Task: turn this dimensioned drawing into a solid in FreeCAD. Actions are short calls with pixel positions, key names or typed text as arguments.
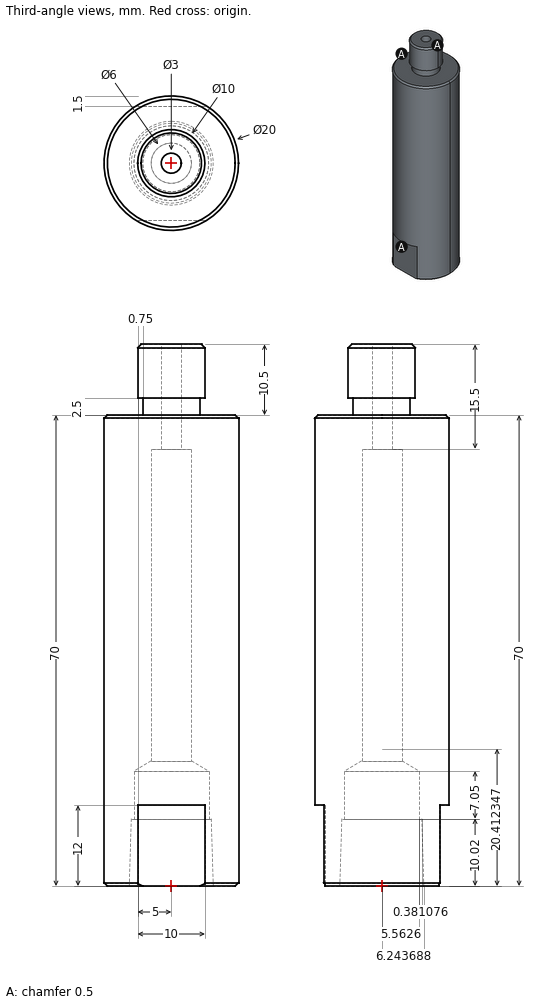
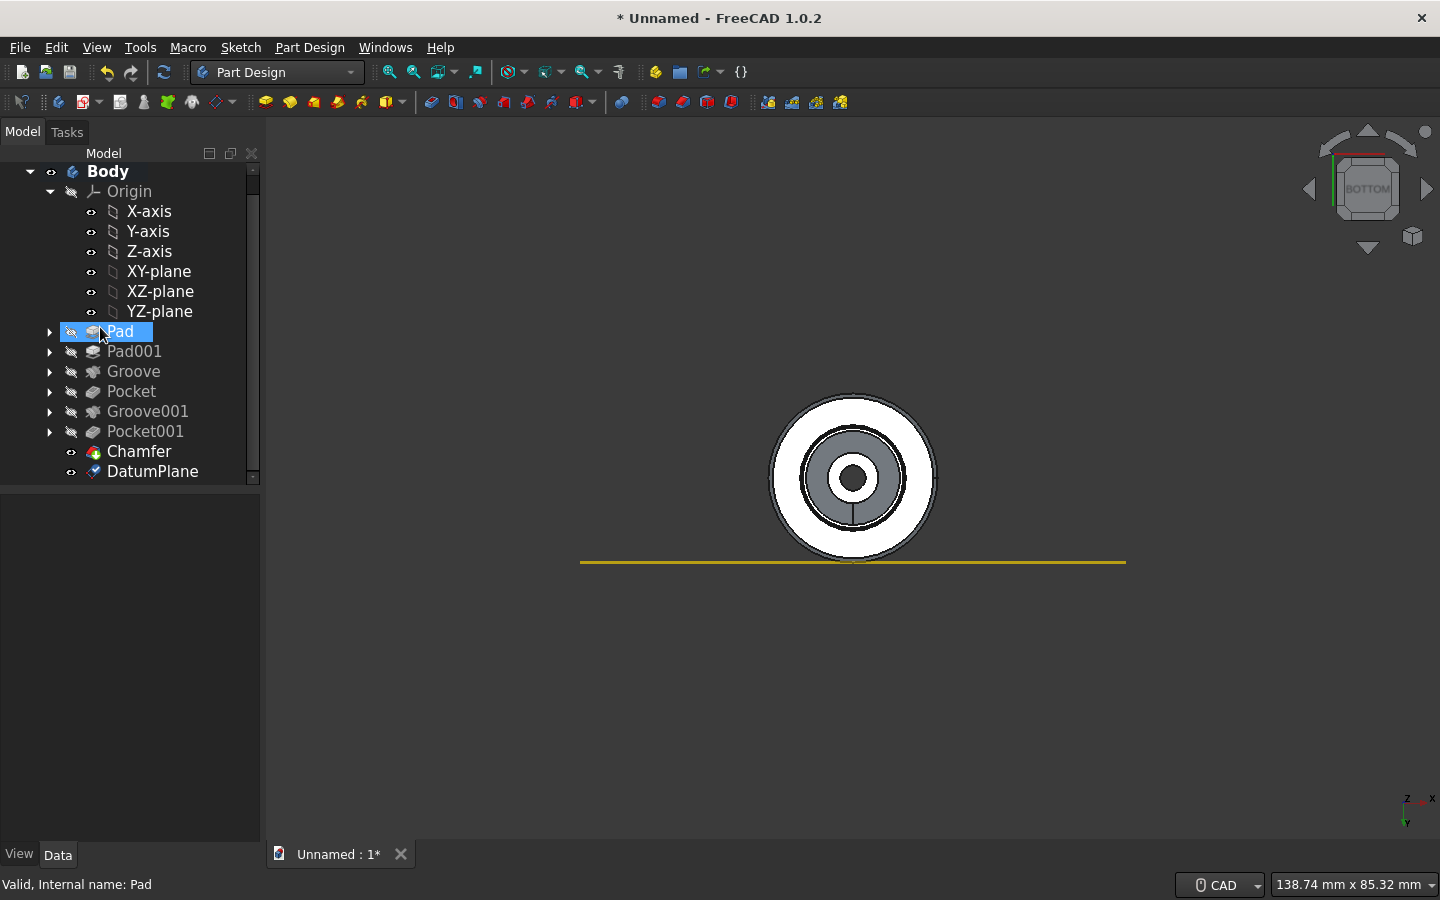
click(116, 472)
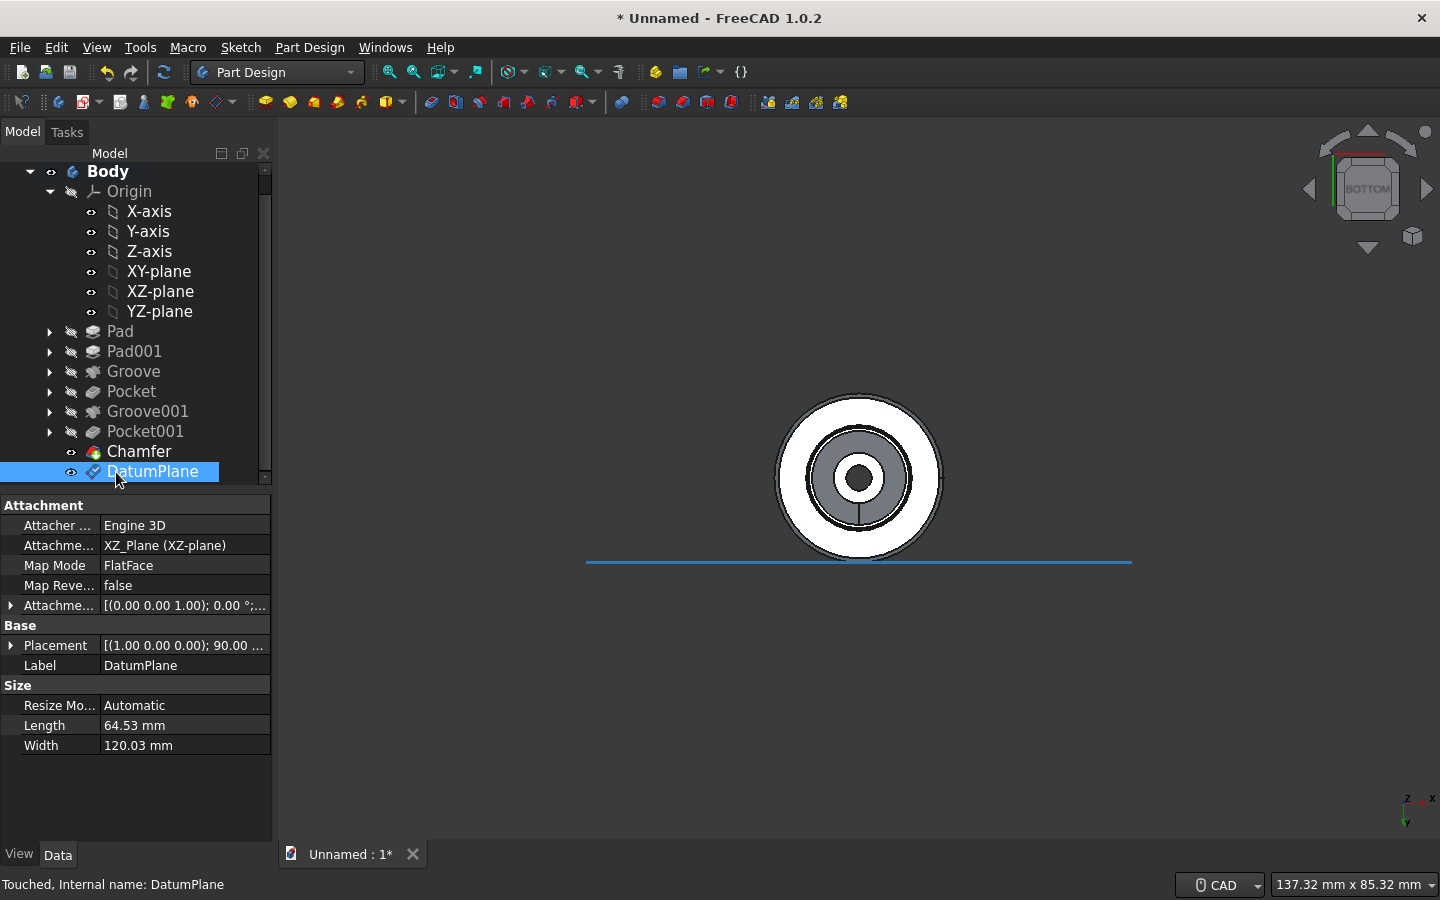
click(84, 102)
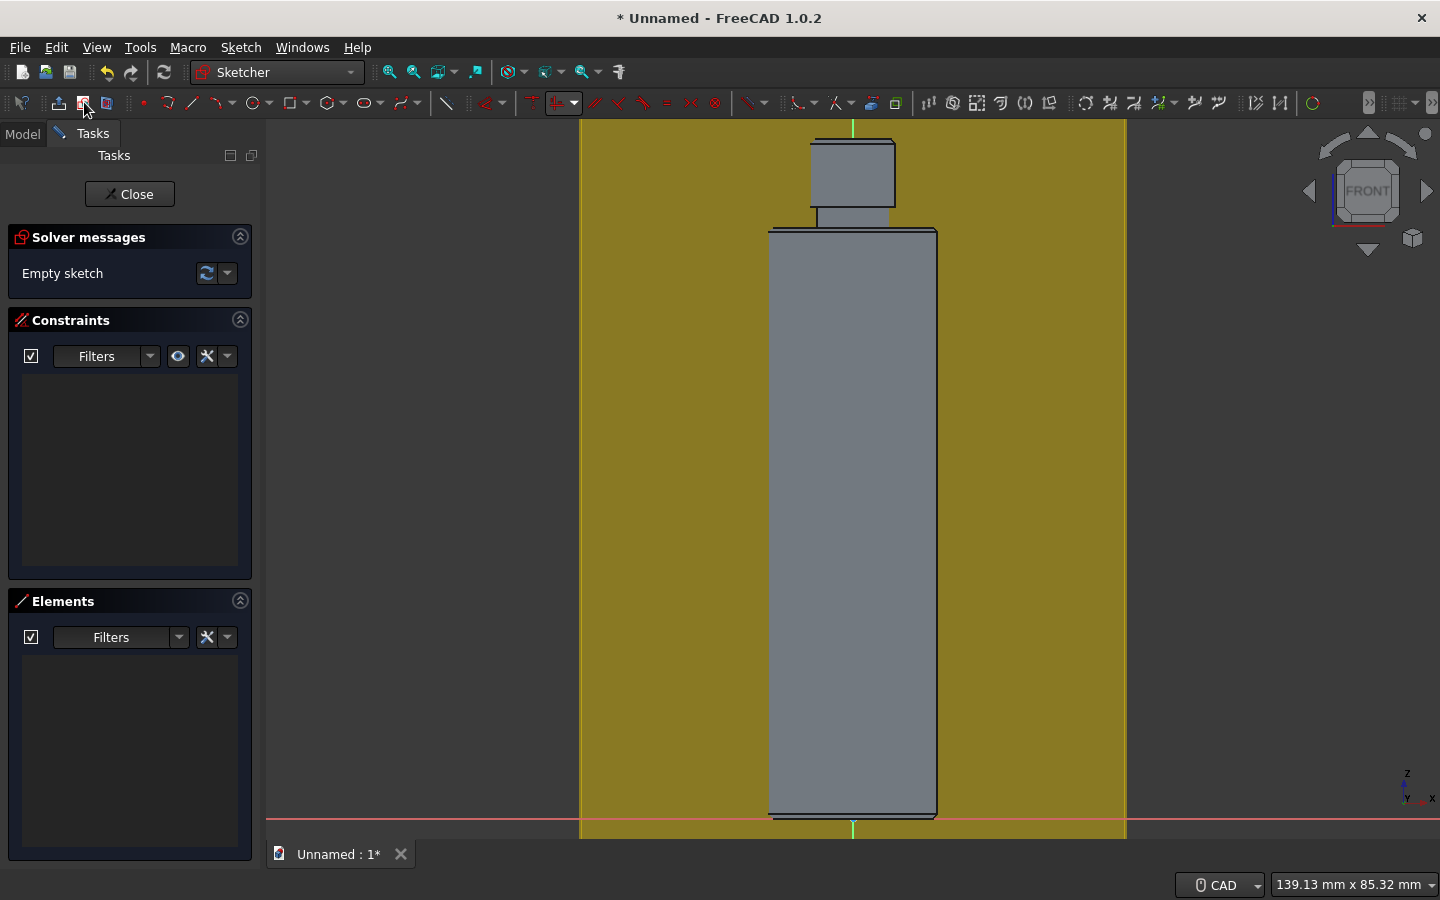
click(108, 104)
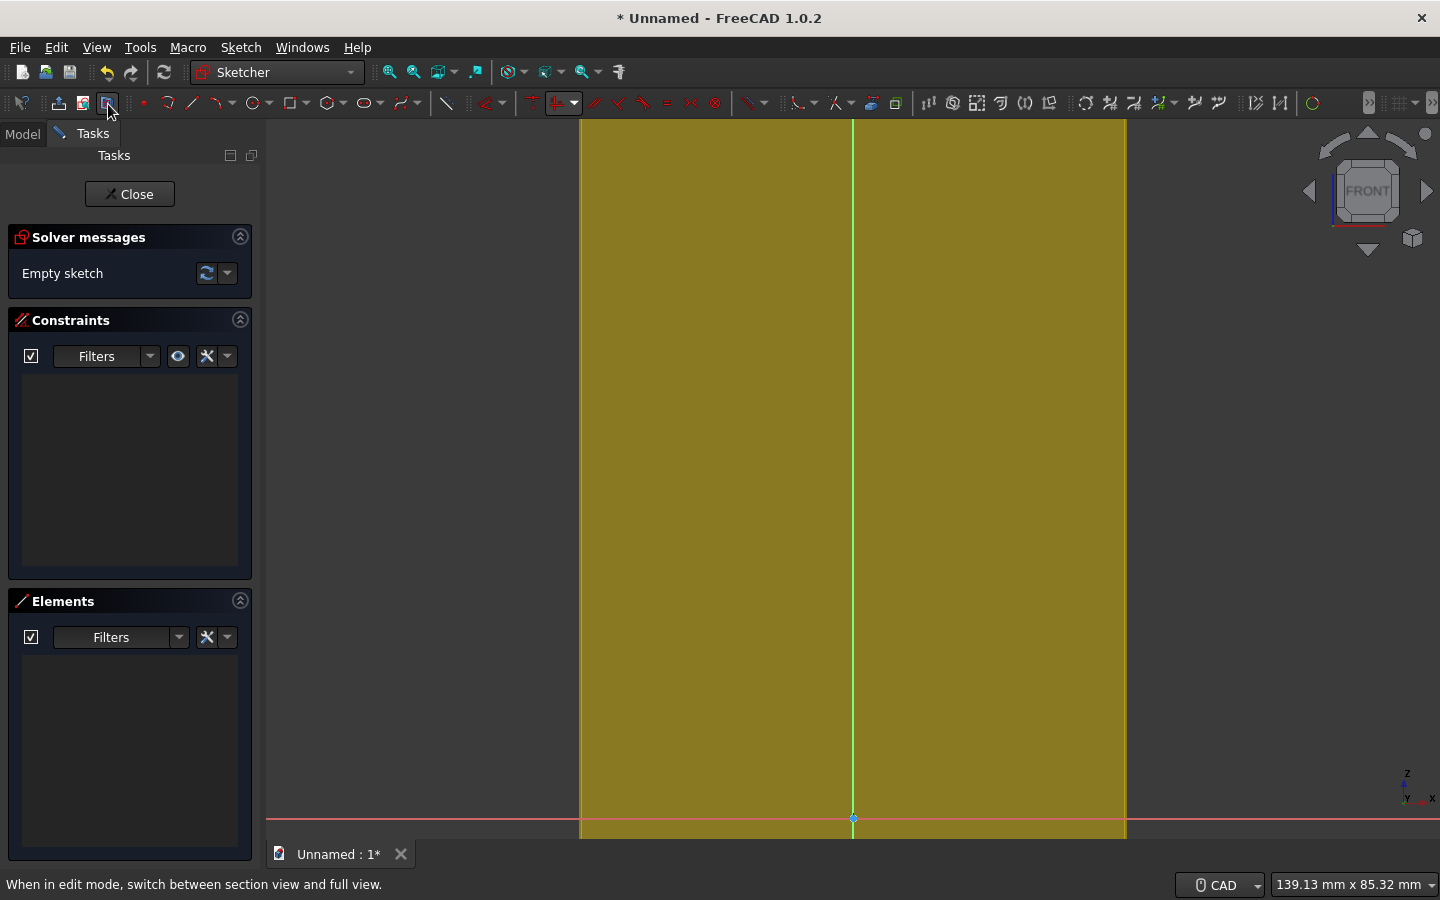
scroll(784, 479, down, 5)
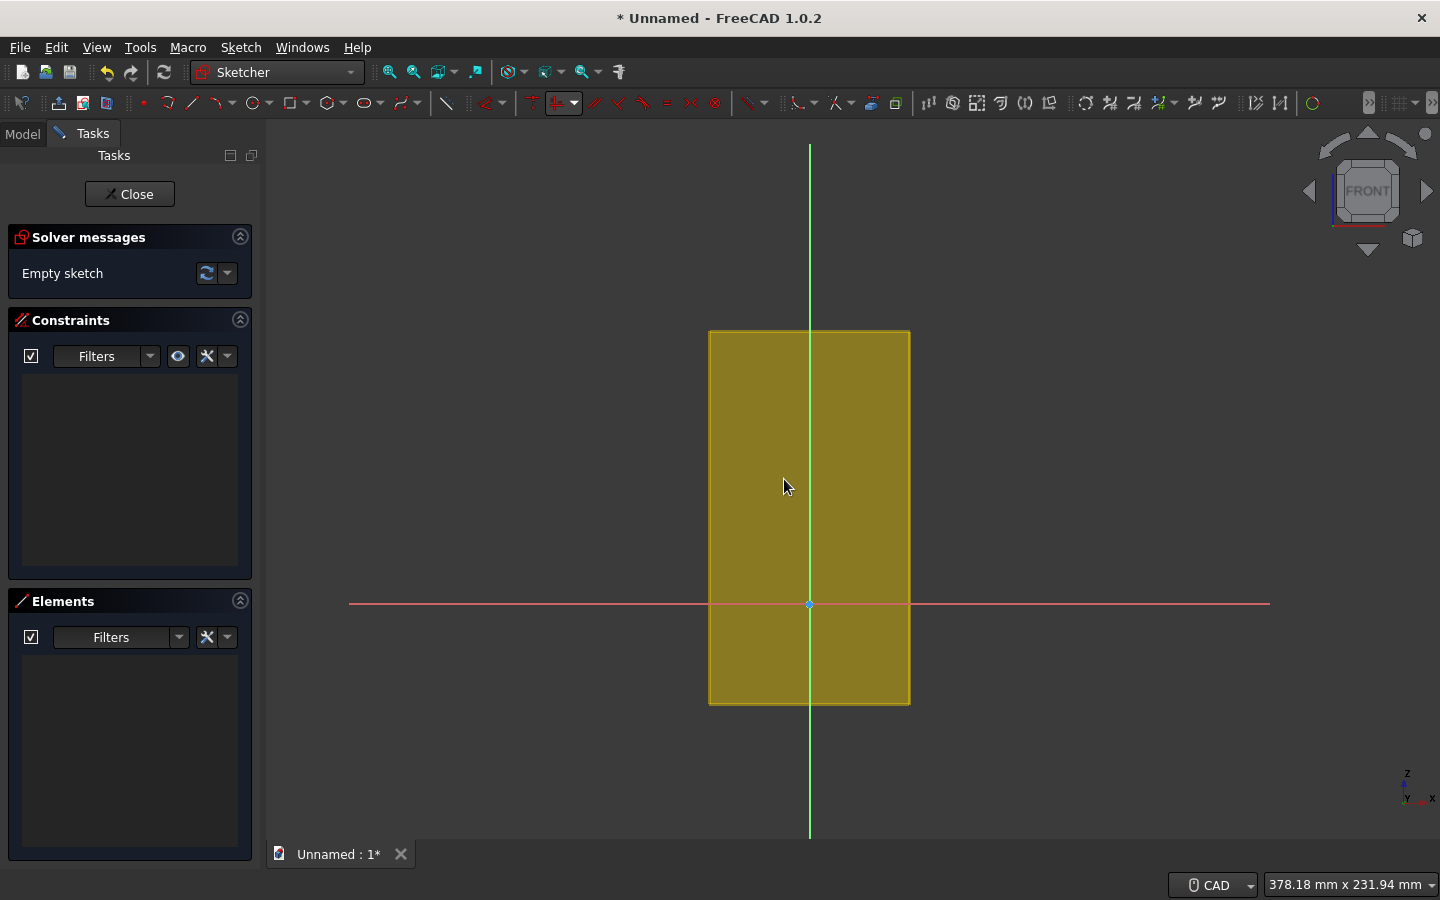
scroll(812, 594, up, 13)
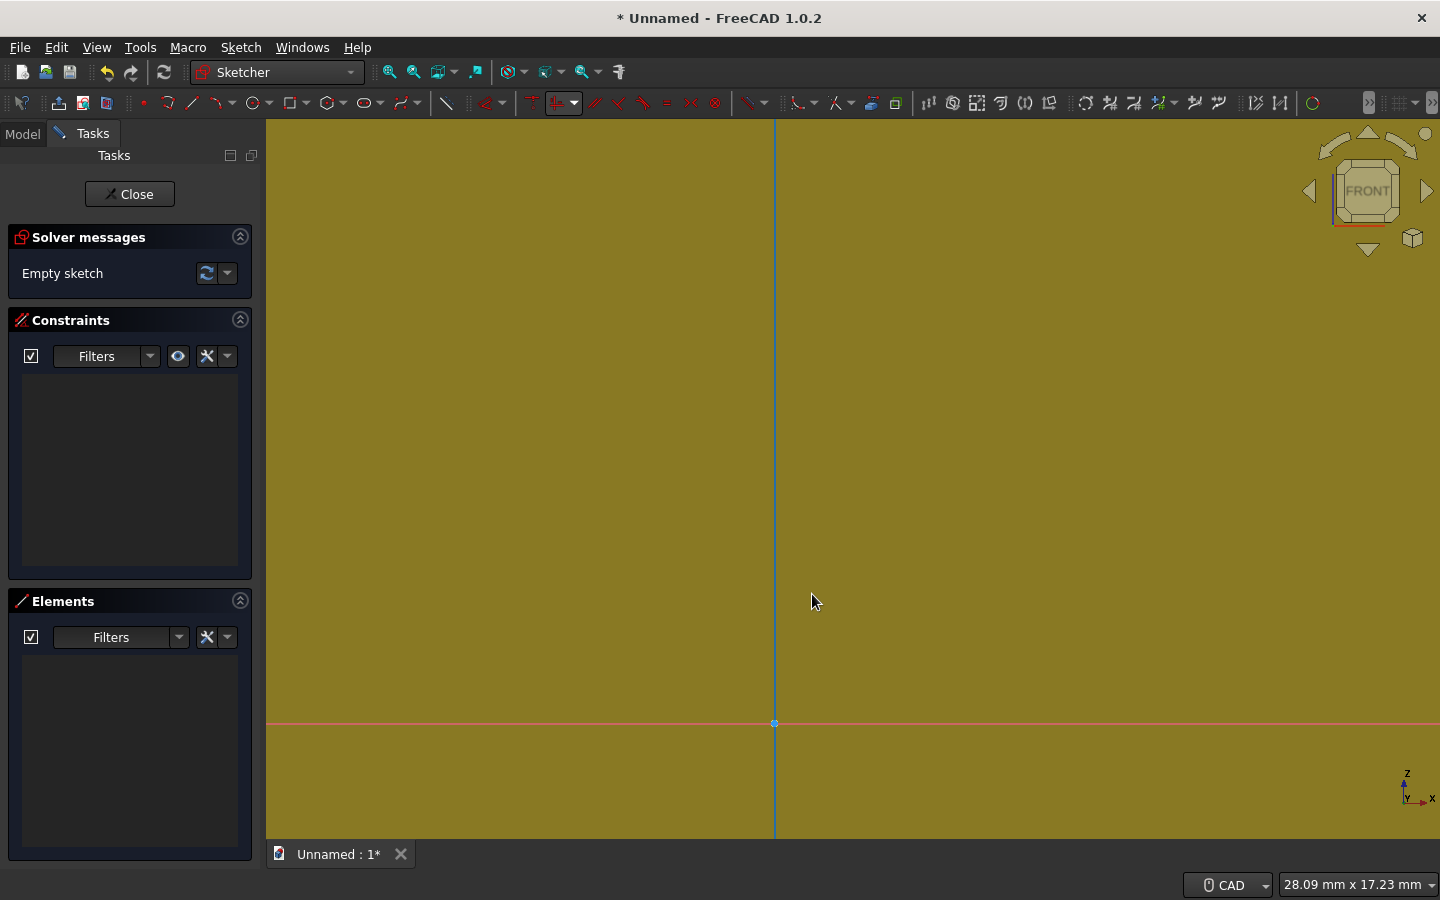
click(290, 104)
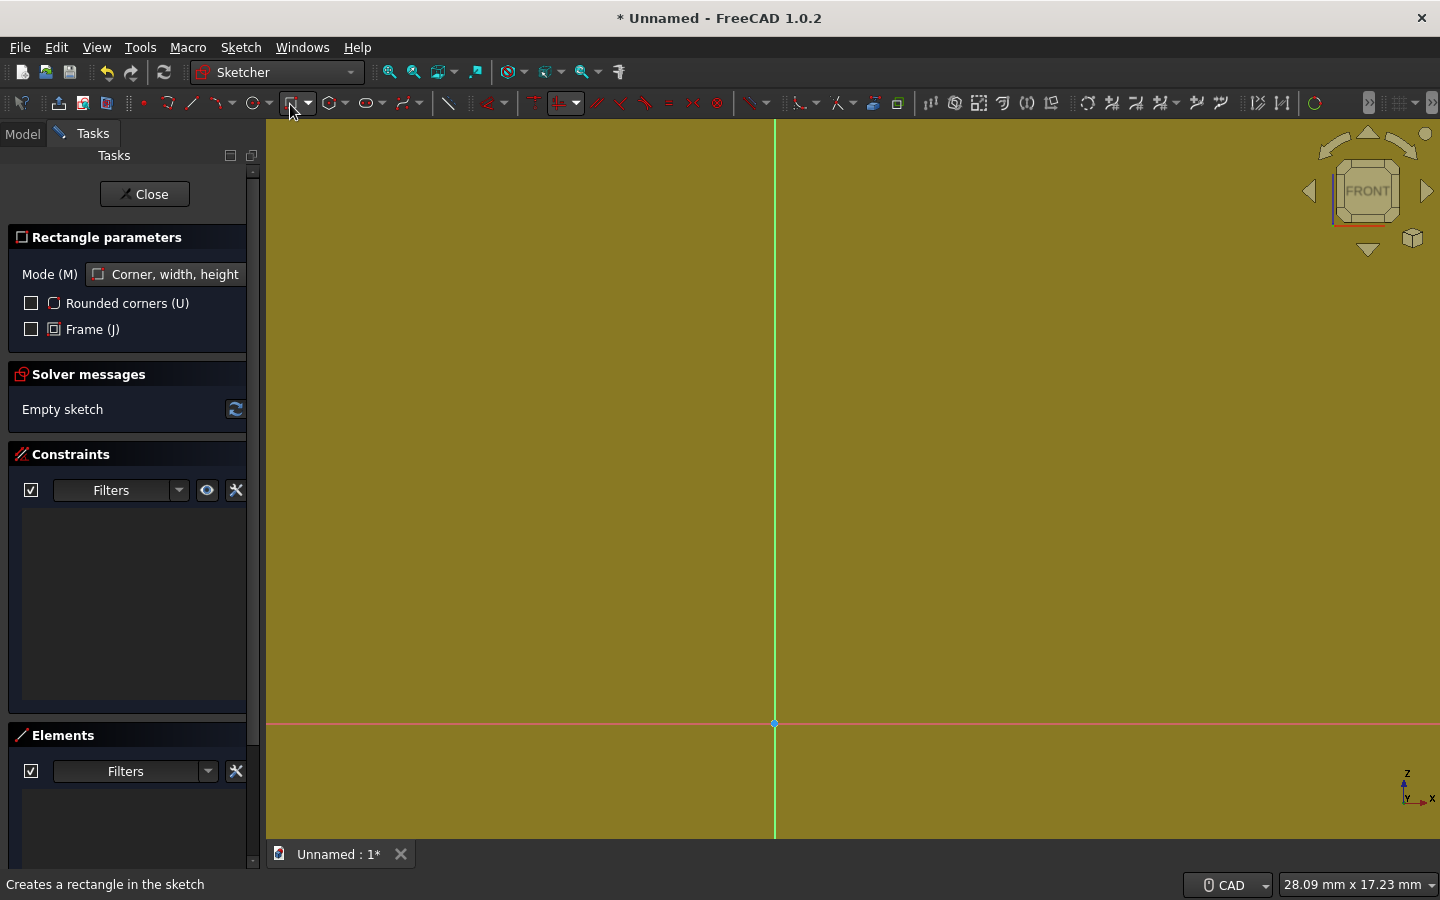
click(566, 222)
click(984, 724)
key(Escape)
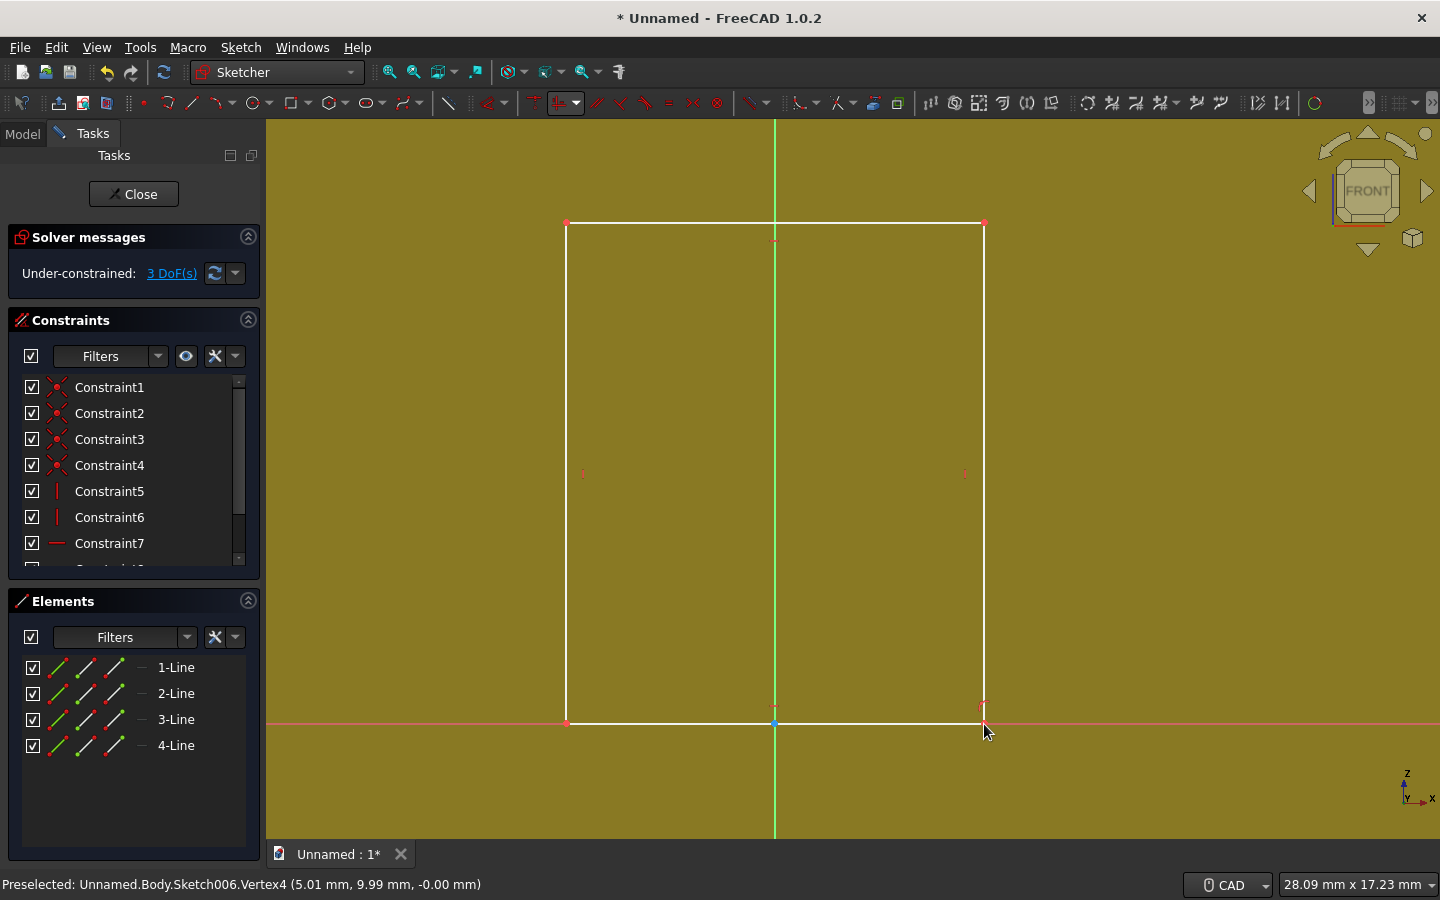
key(d)